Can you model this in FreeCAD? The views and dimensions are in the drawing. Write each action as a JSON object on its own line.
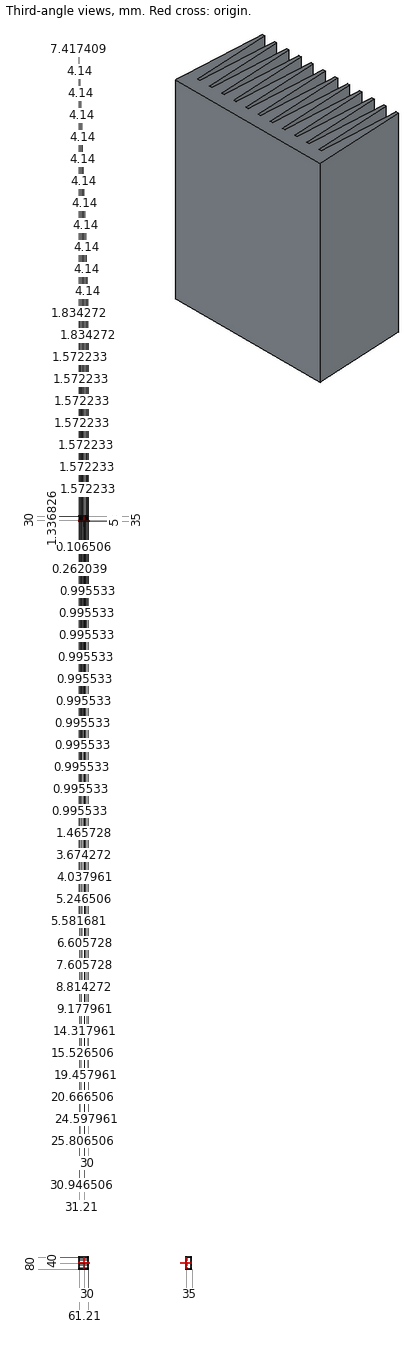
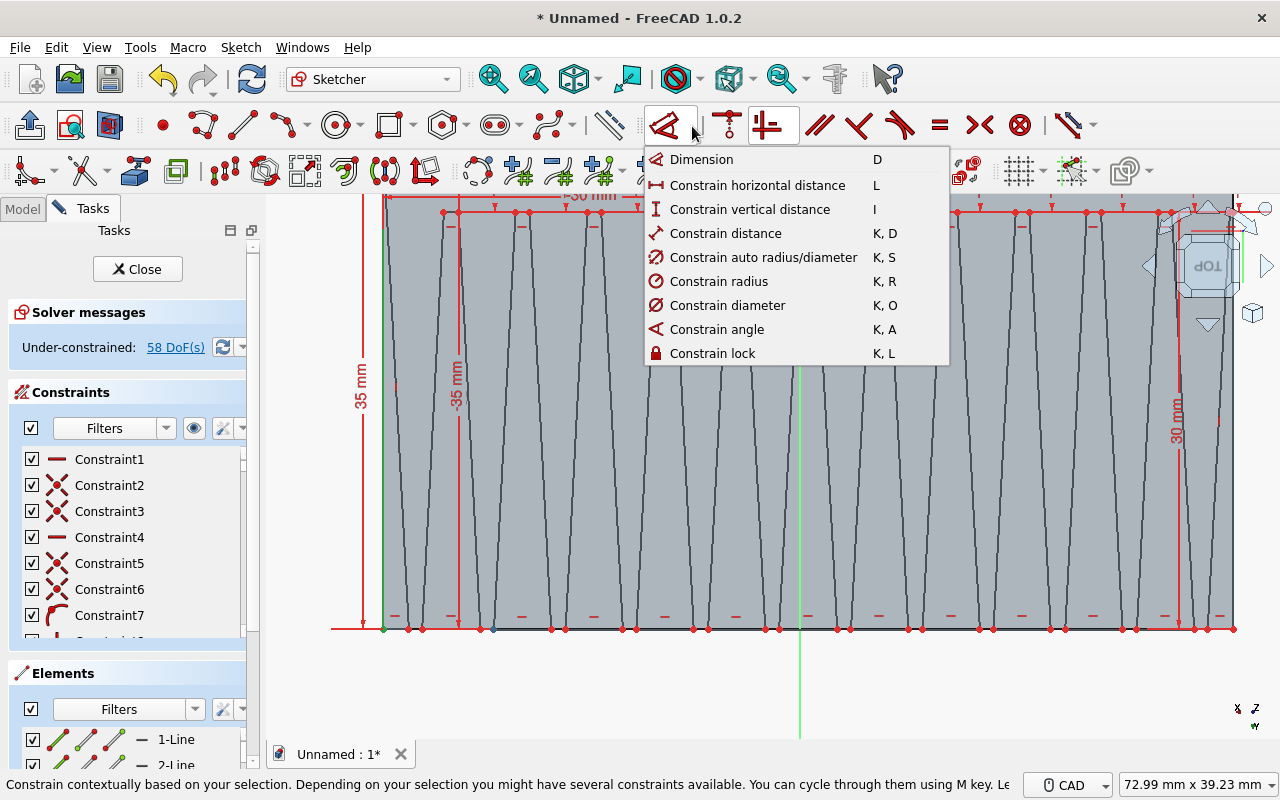
{"action": "left_click", "coordinate": [797, 209]}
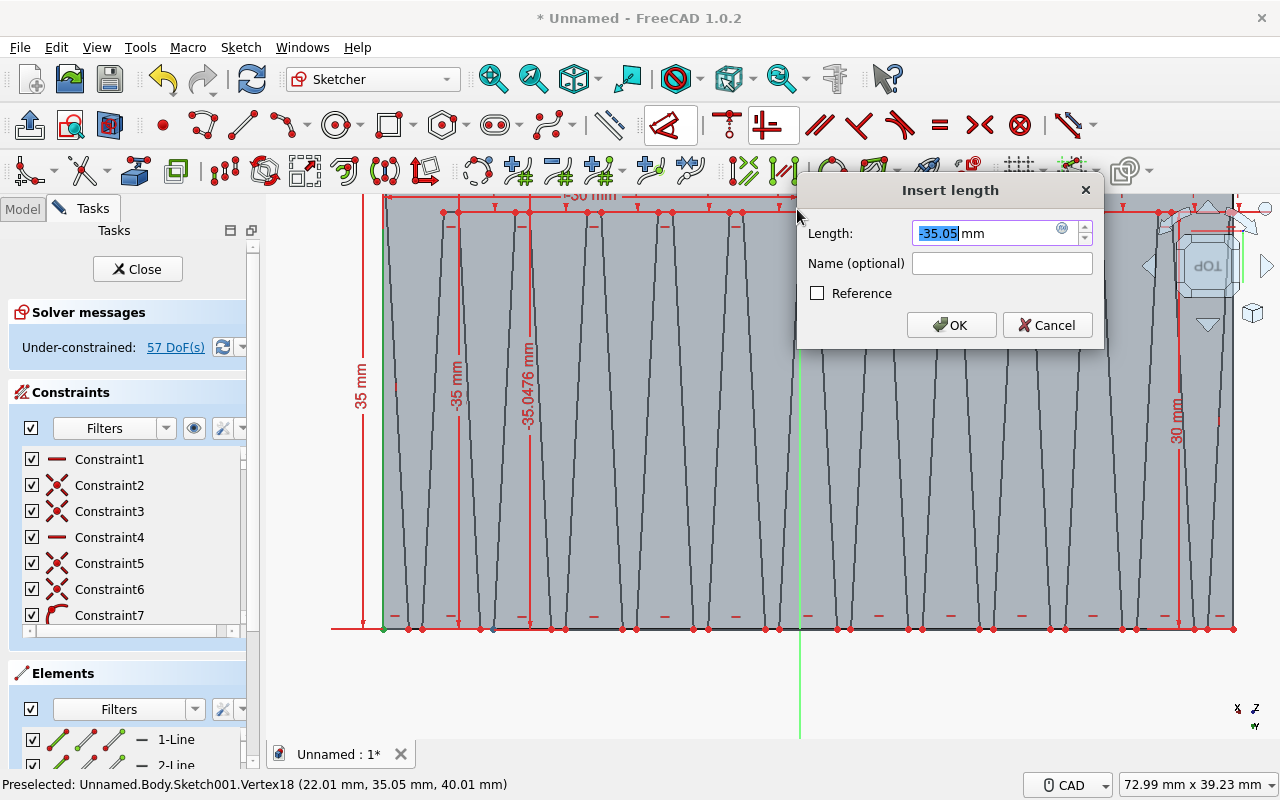
{"action": "type", "text": "-35"}
{"action": "key", "text": "Return"}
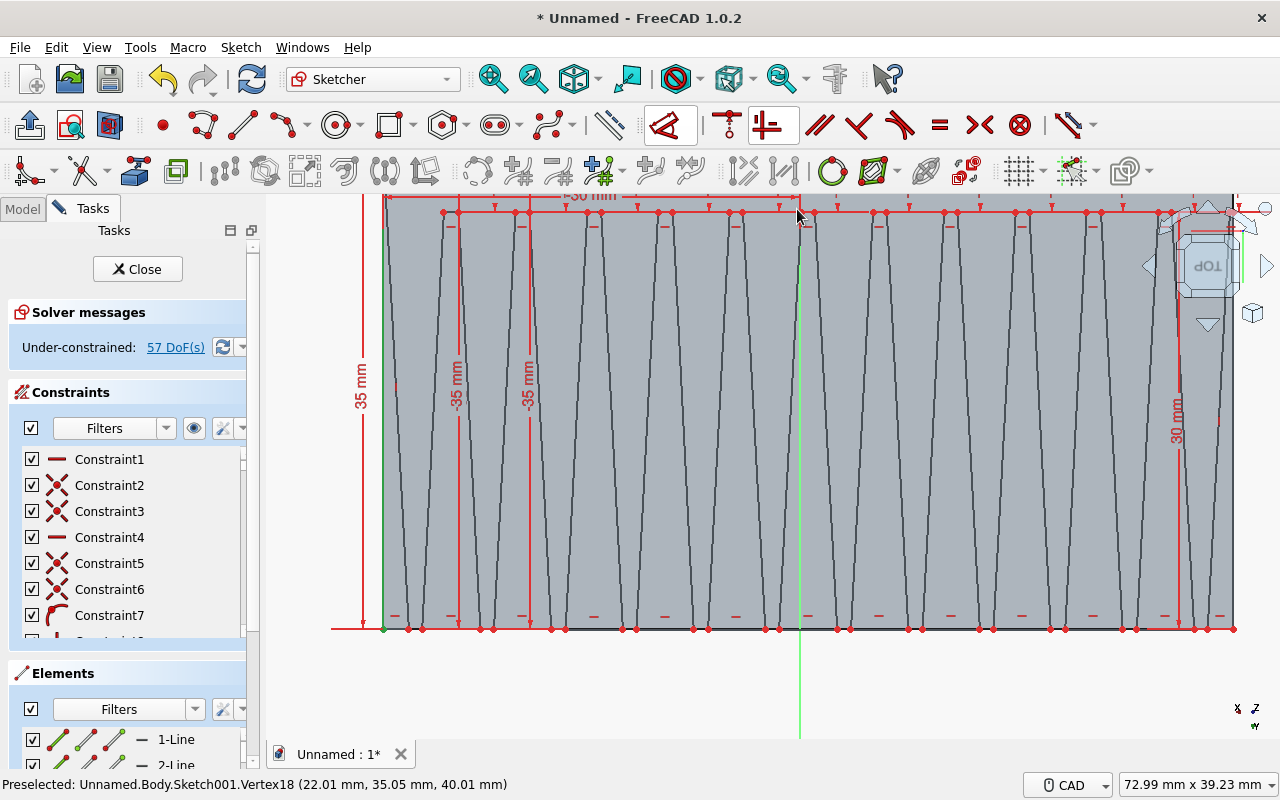
{"action": "left_click", "coordinate": [566, 630]}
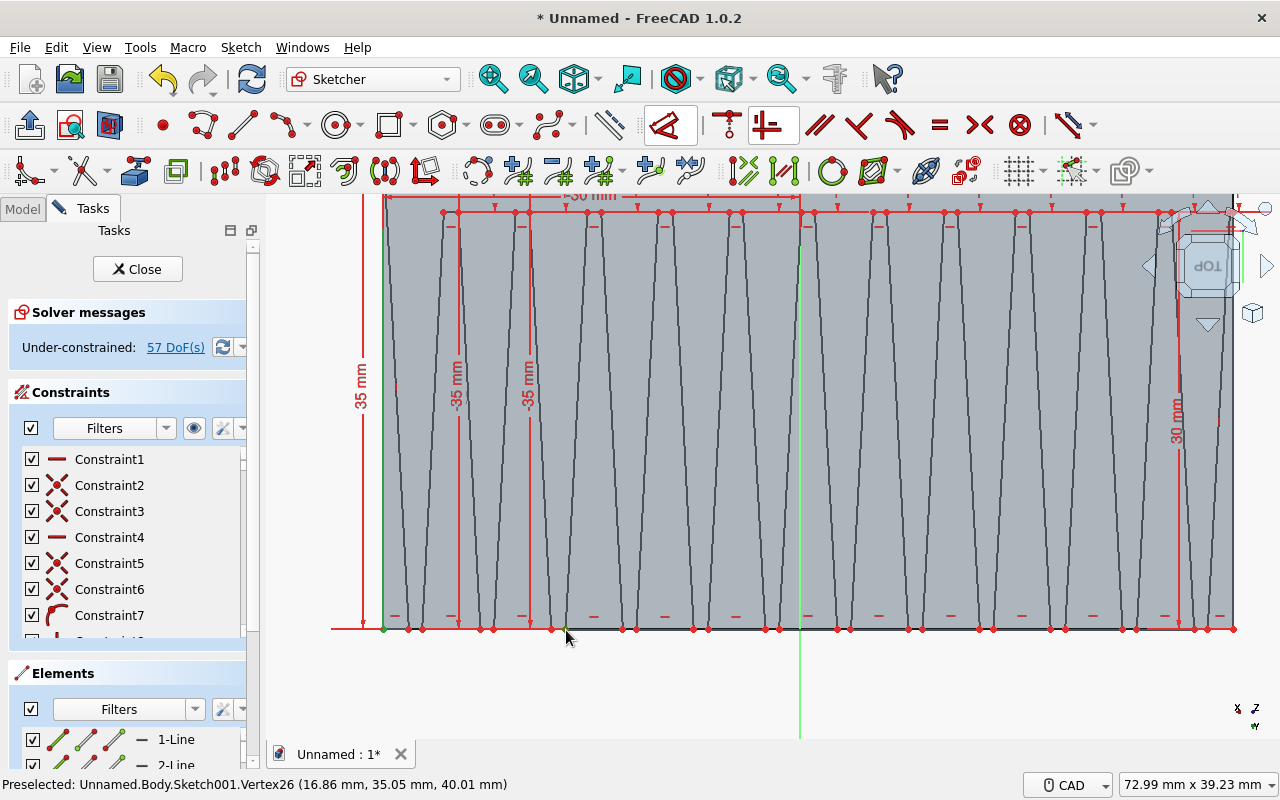
{"action": "left_click", "coordinate": [692, 126]}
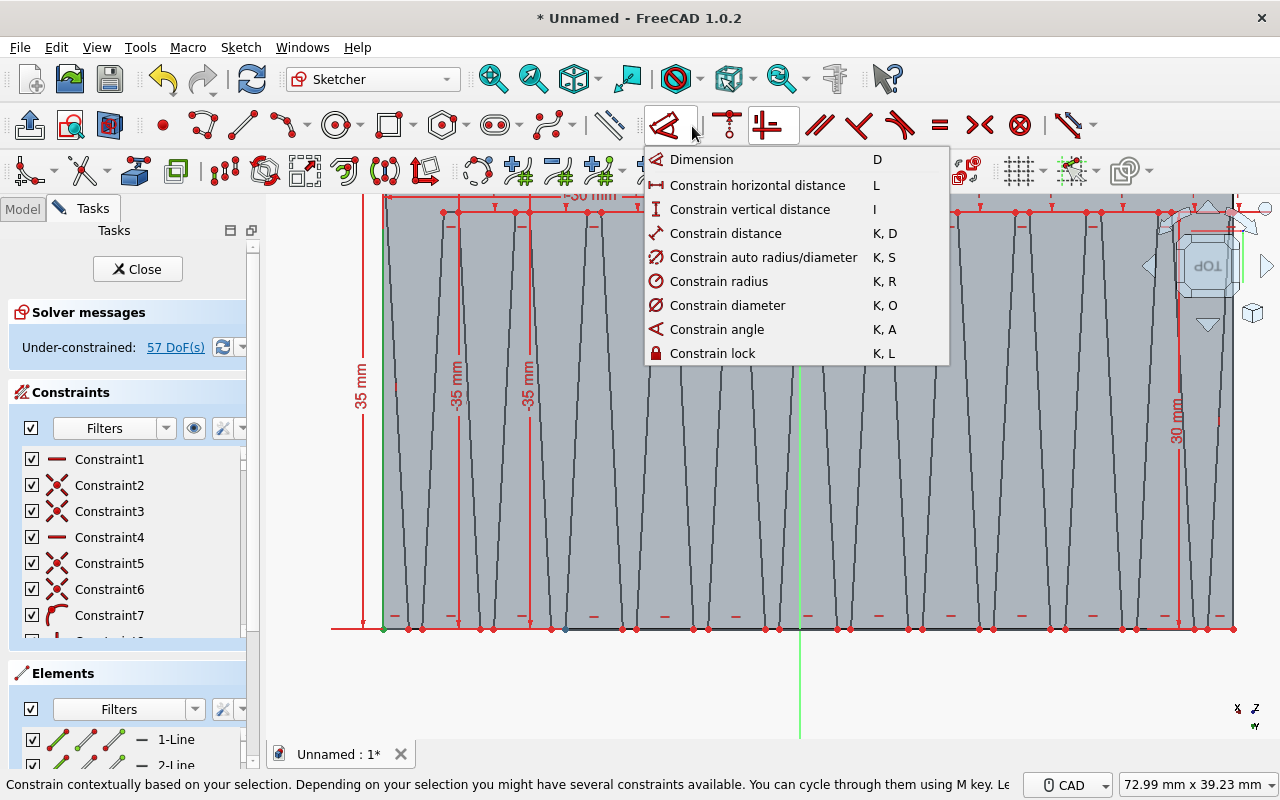
{"action": "left_click", "coordinate": [797, 209]}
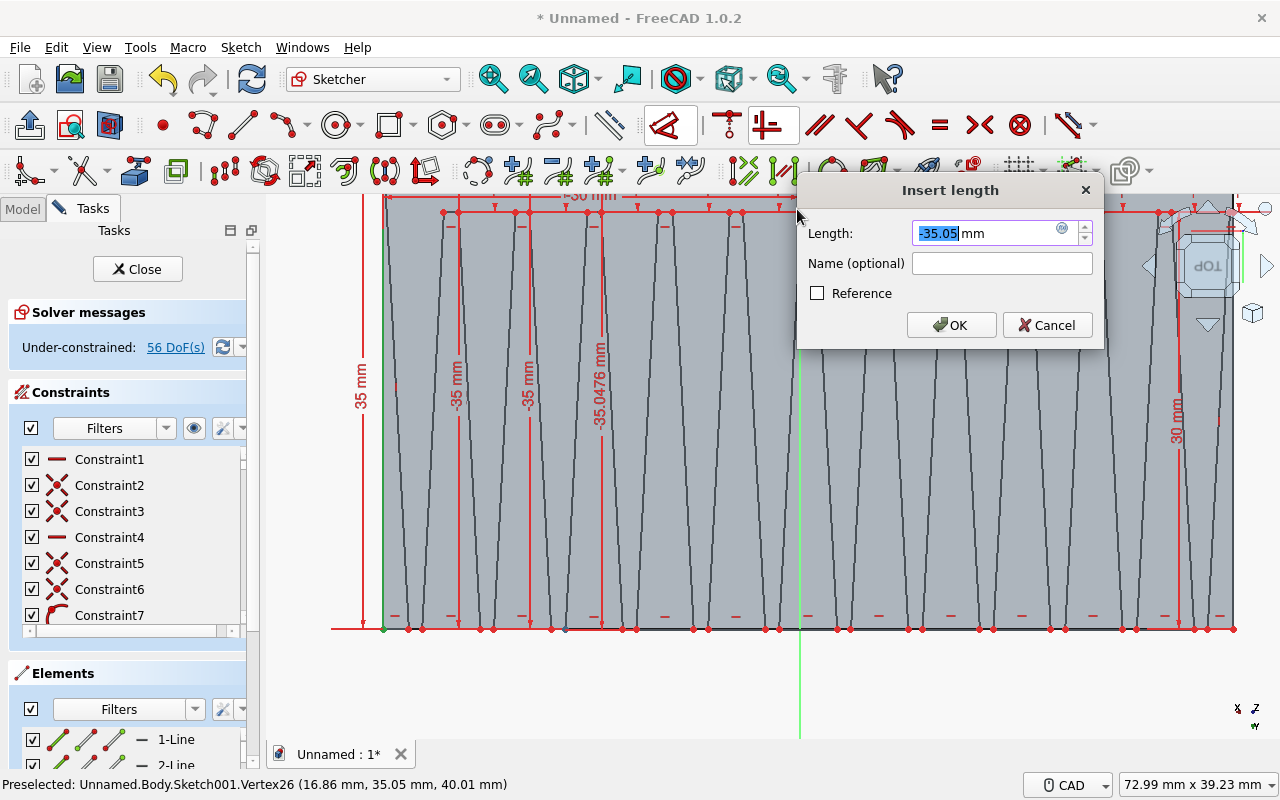
{"action": "type", "text": "-35"}
{"action": "key", "text": "Return"}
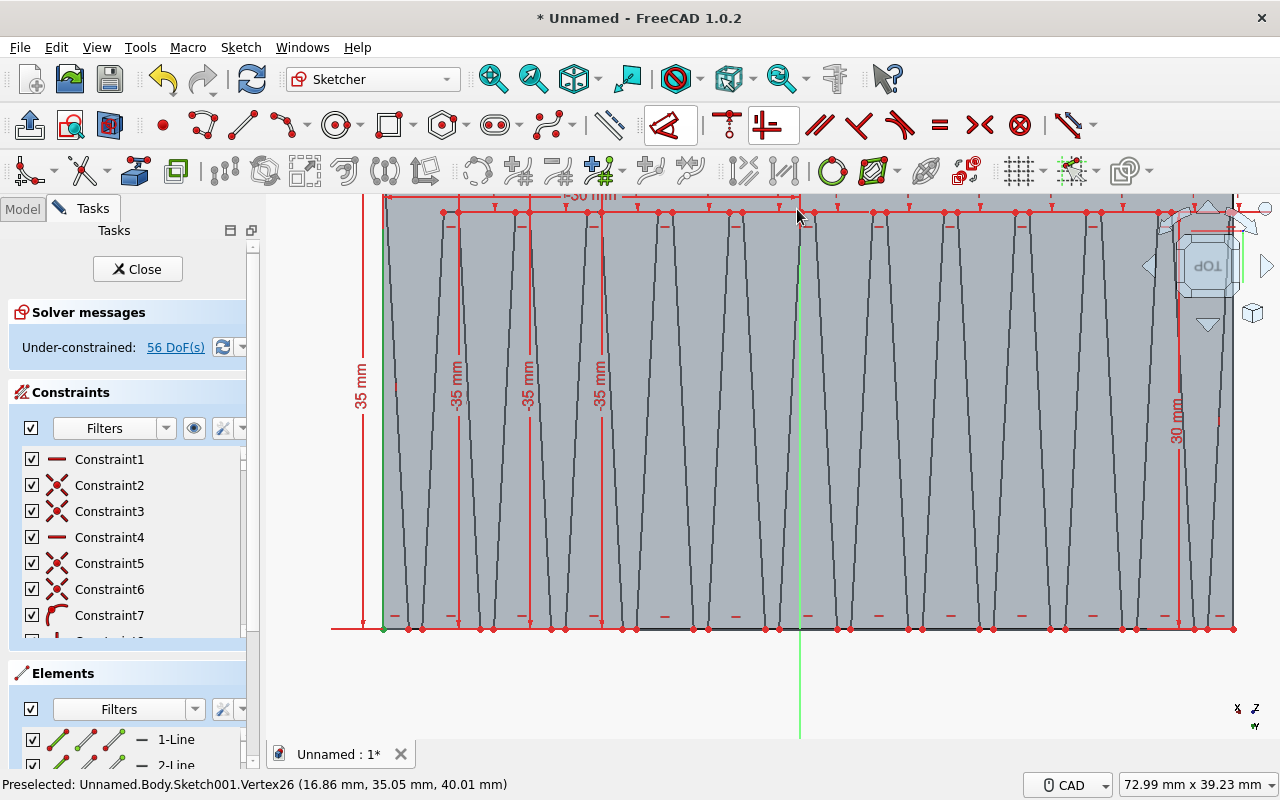
{"action": "left_click", "coordinate": [636, 630]}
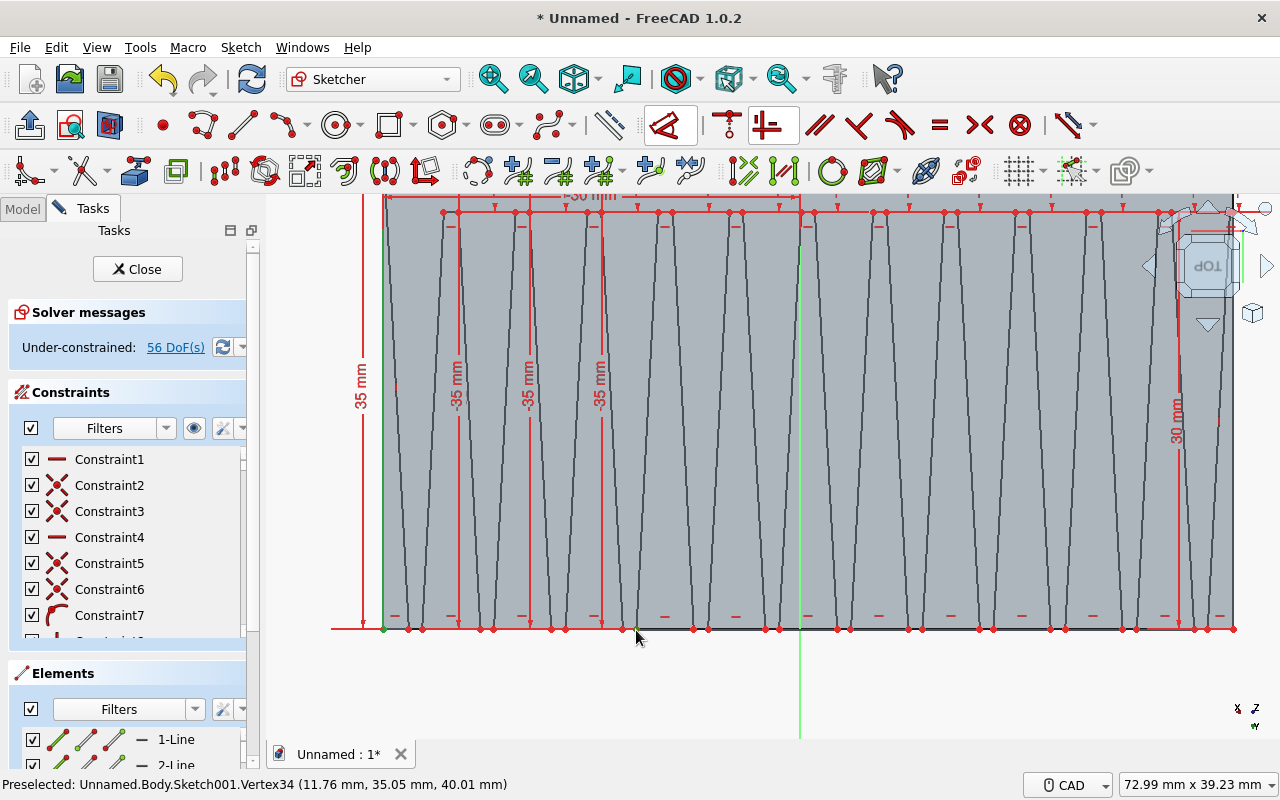
{"action": "key", "text": "i"}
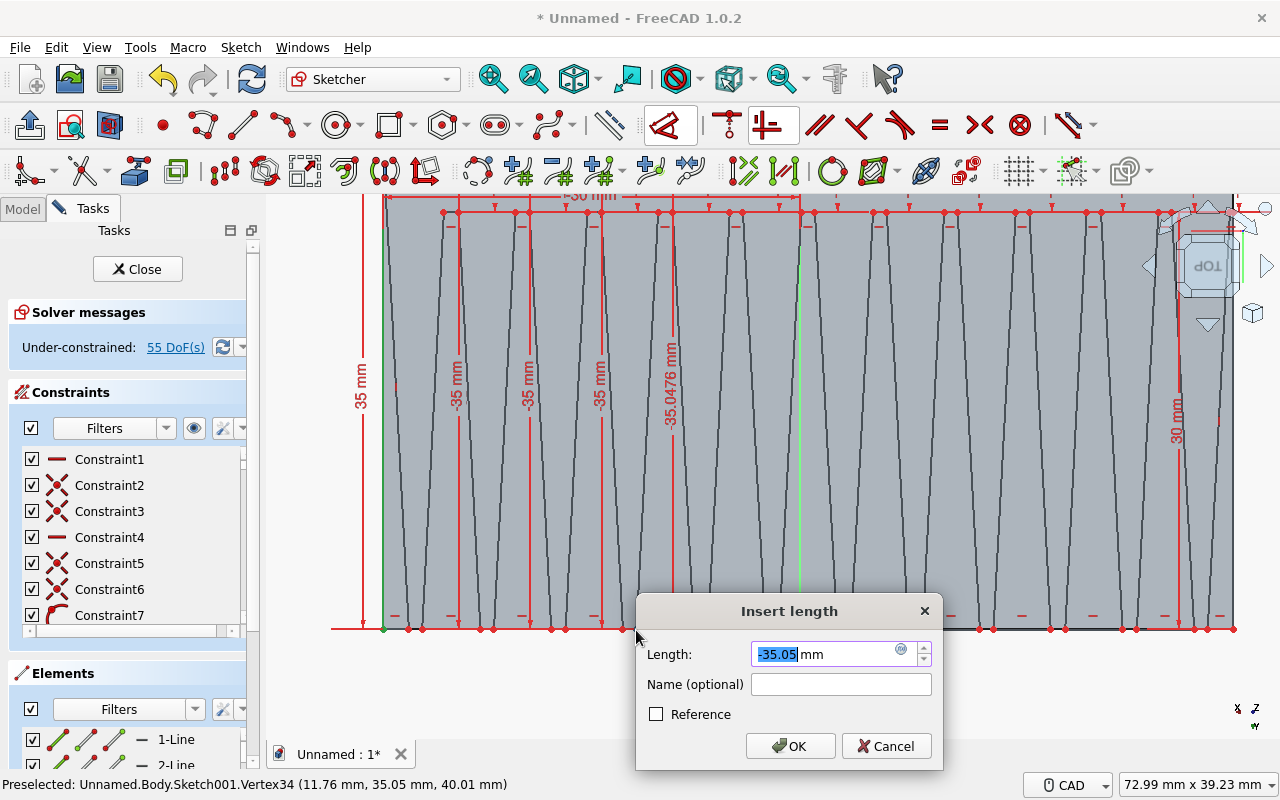
{"action": "type", "text": "-35"}
{"action": "key", "text": "Return"}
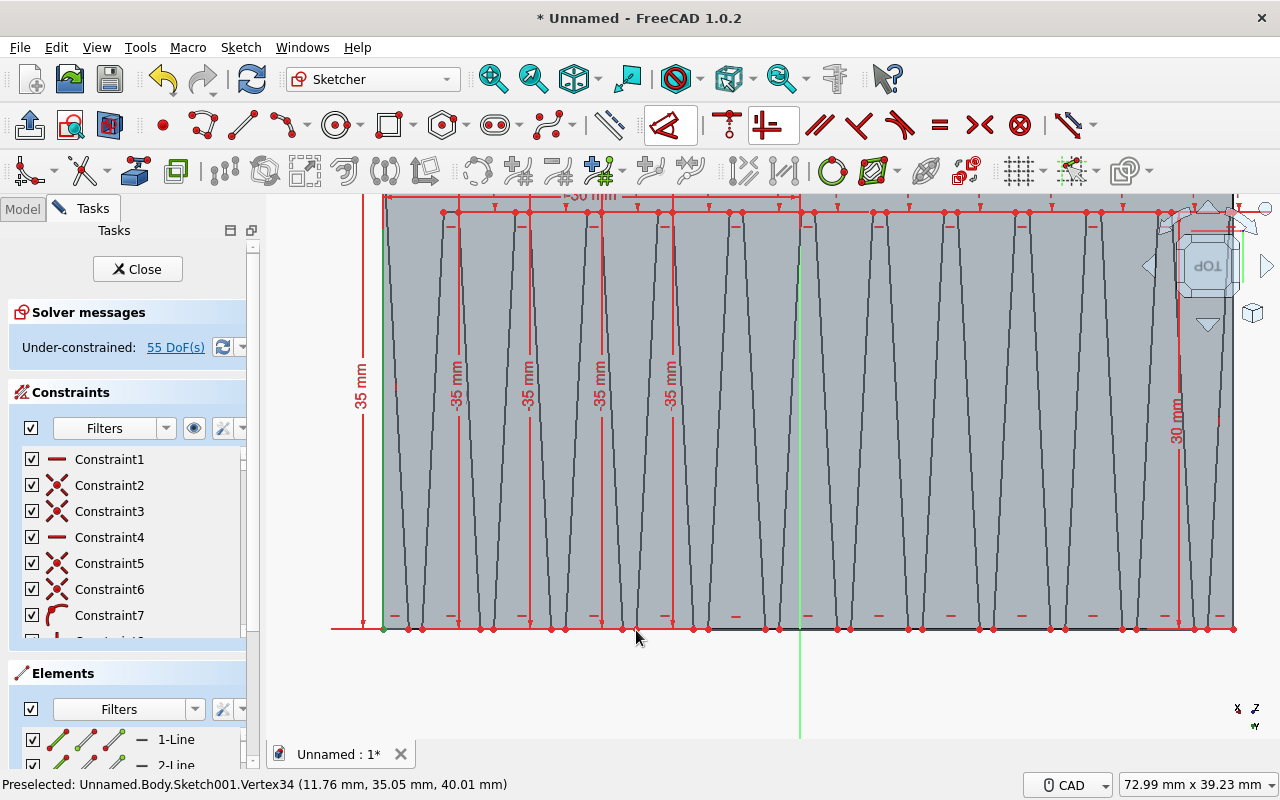
{"action": "left_click", "coordinate": [708, 630]}